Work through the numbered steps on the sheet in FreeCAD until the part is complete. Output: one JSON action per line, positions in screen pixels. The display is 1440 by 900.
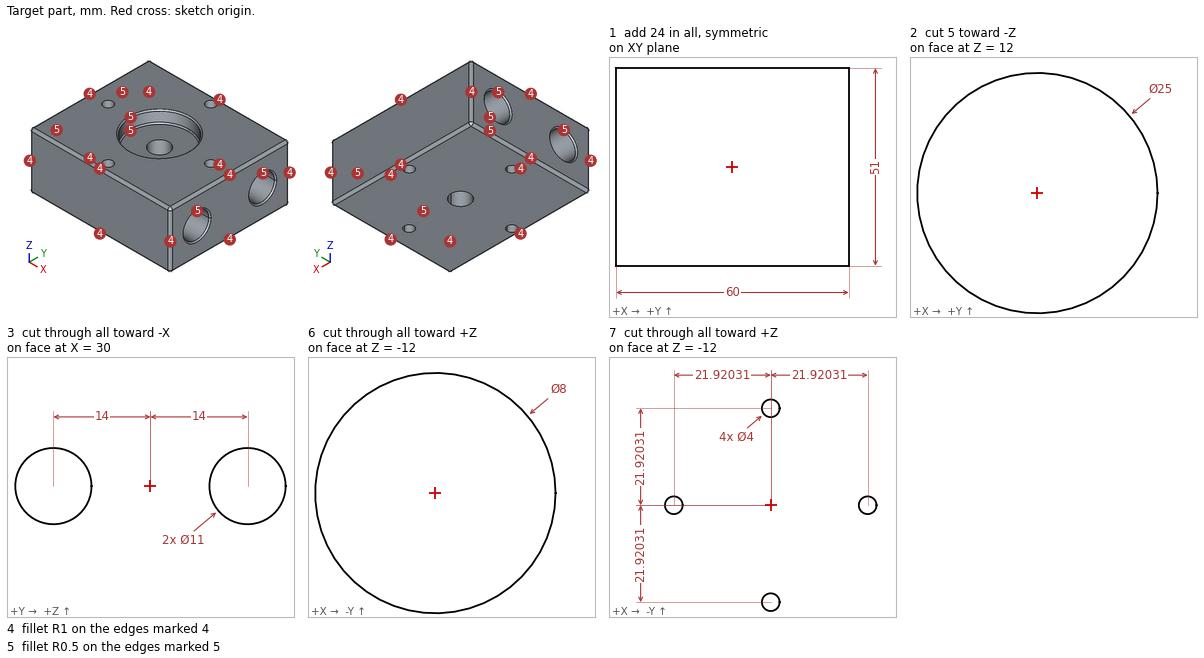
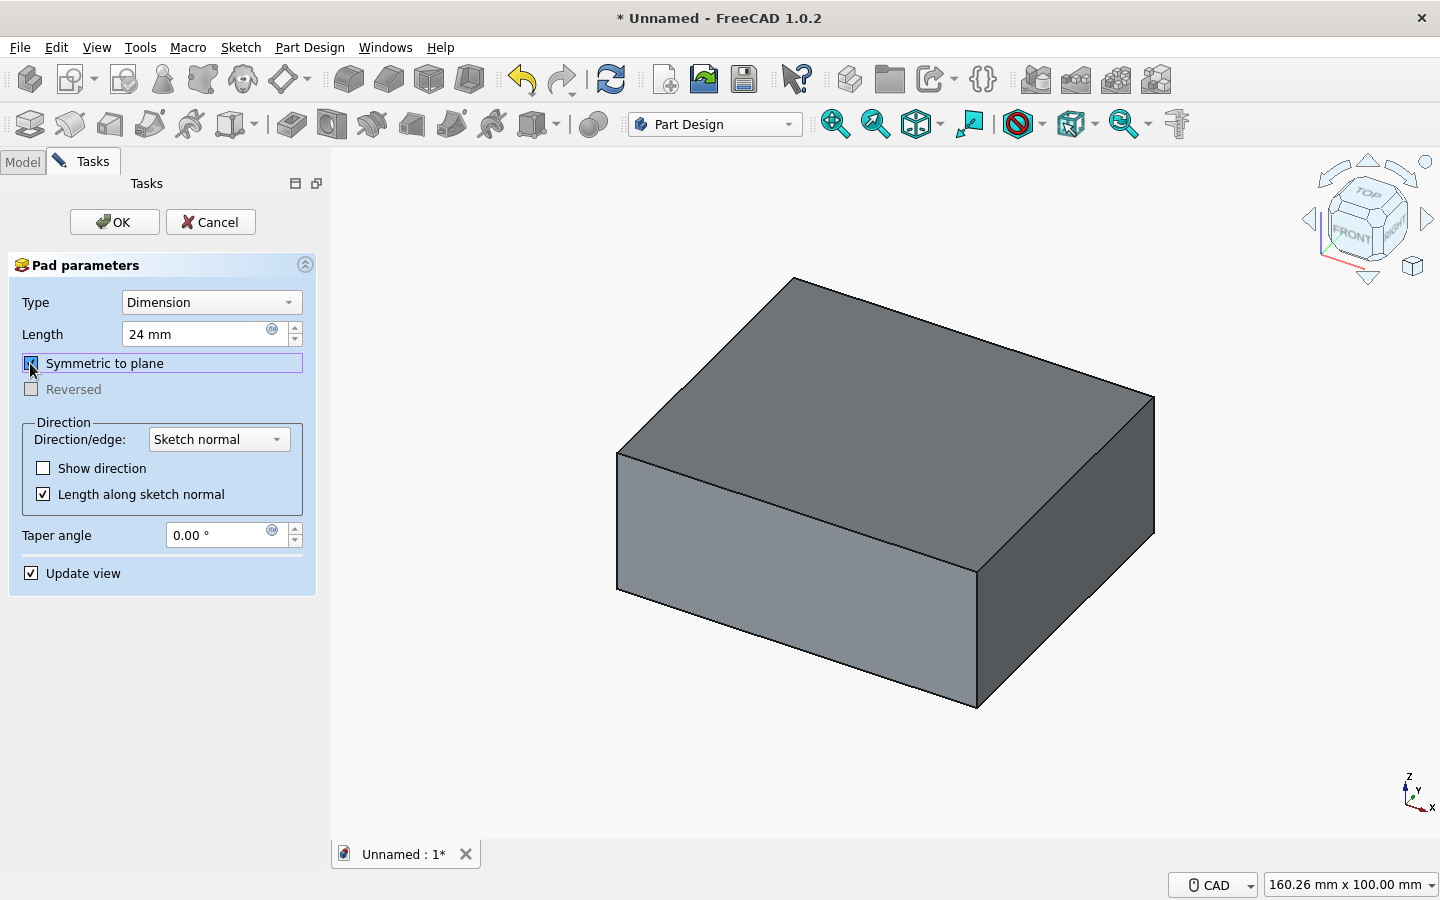
{"action": "left_click", "coordinate": [115, 222]}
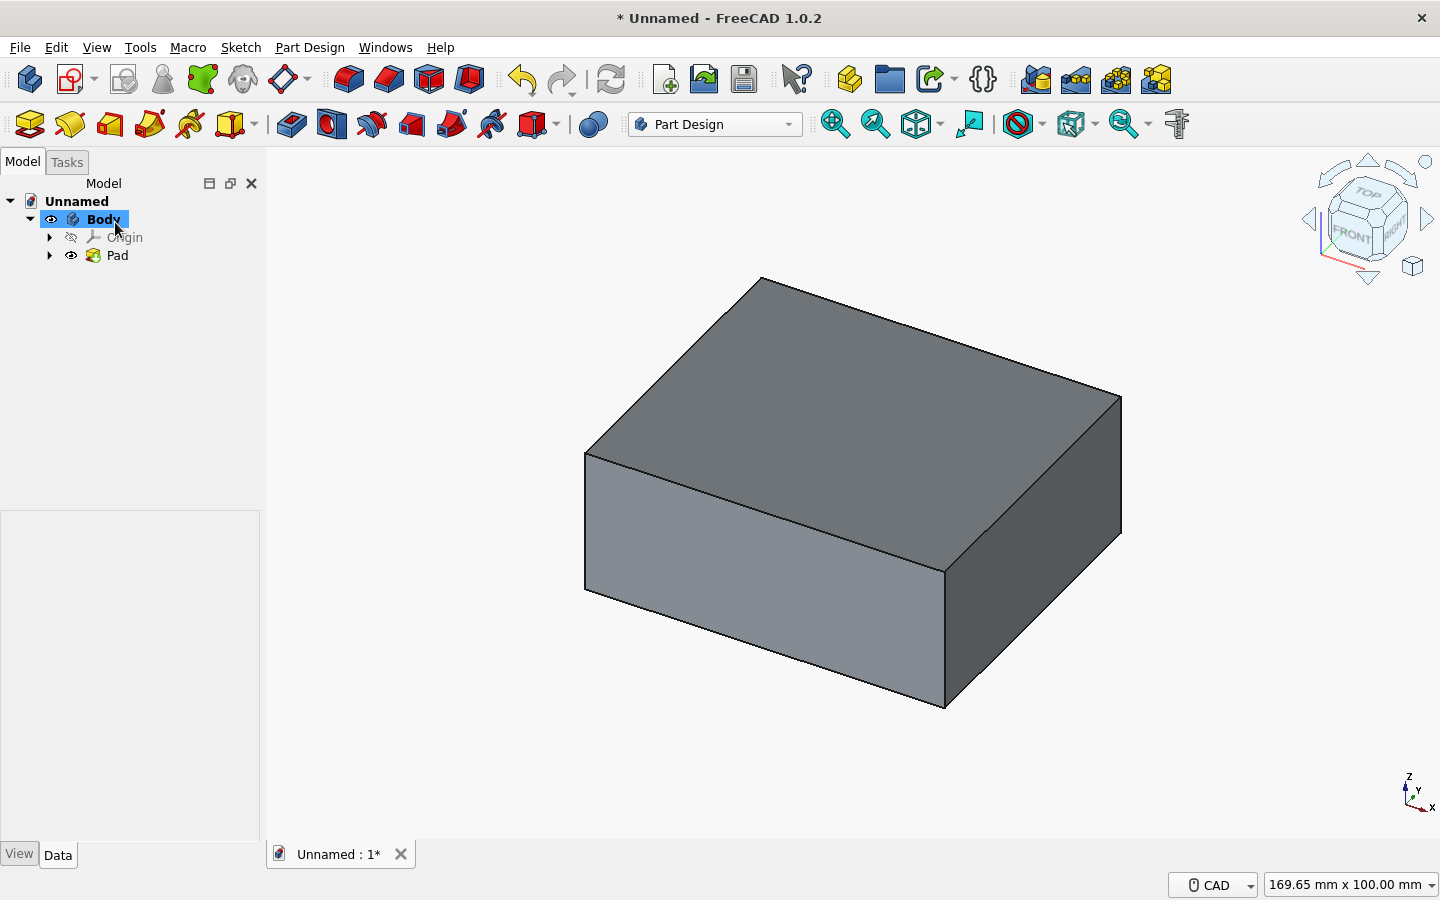
{"action": "left_click", "coordinate": [853, 424]}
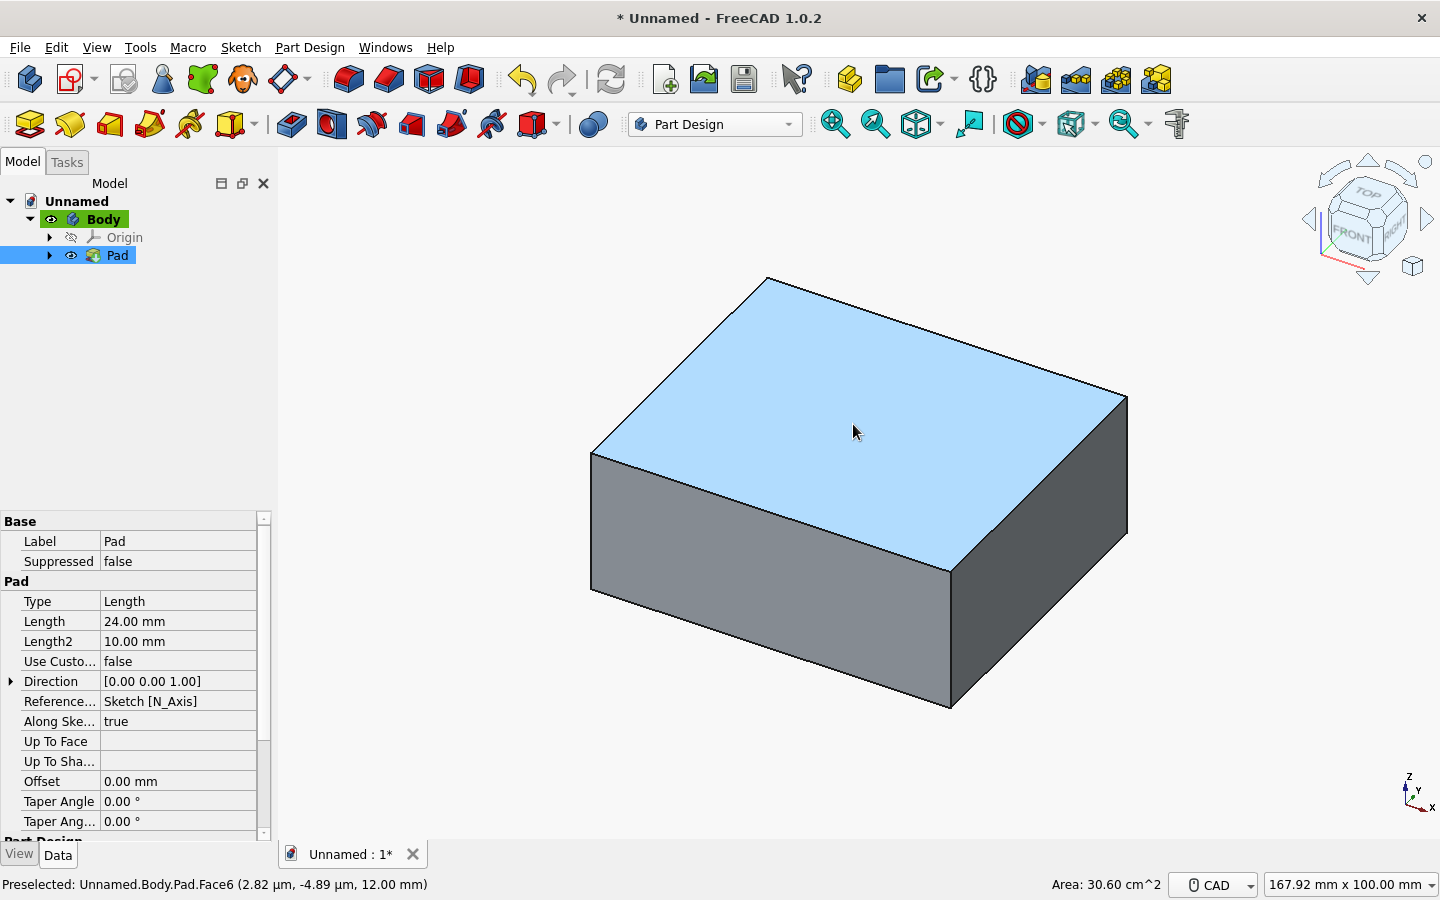
{"action": "left_click", "coordinate": [70, 80]}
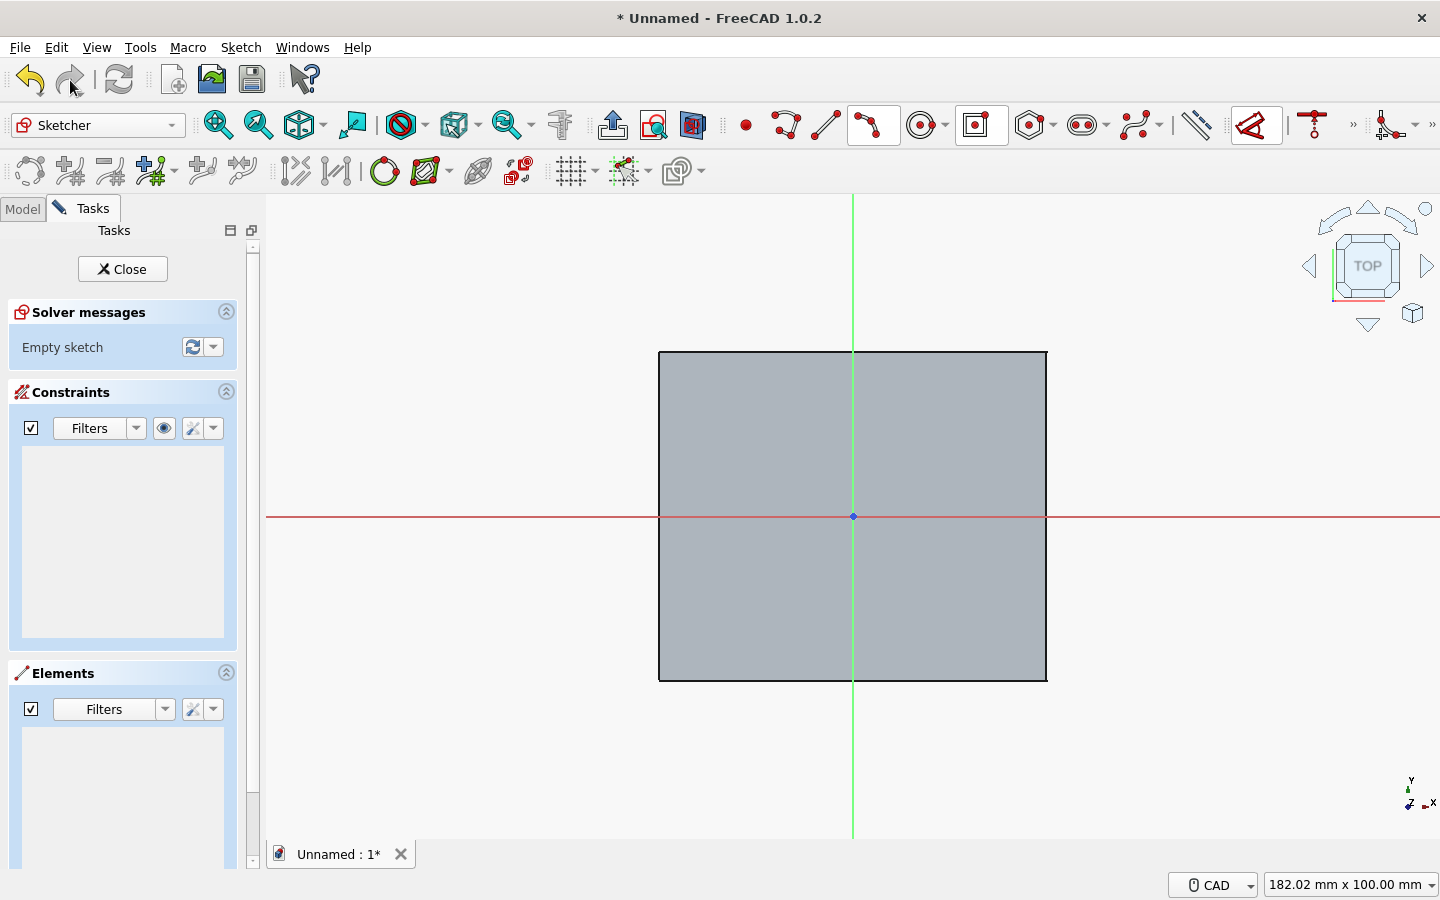
{"action": "scroll", "coordinate": [893, 516], "scroll_direction": "up", "scroll_amount": 5}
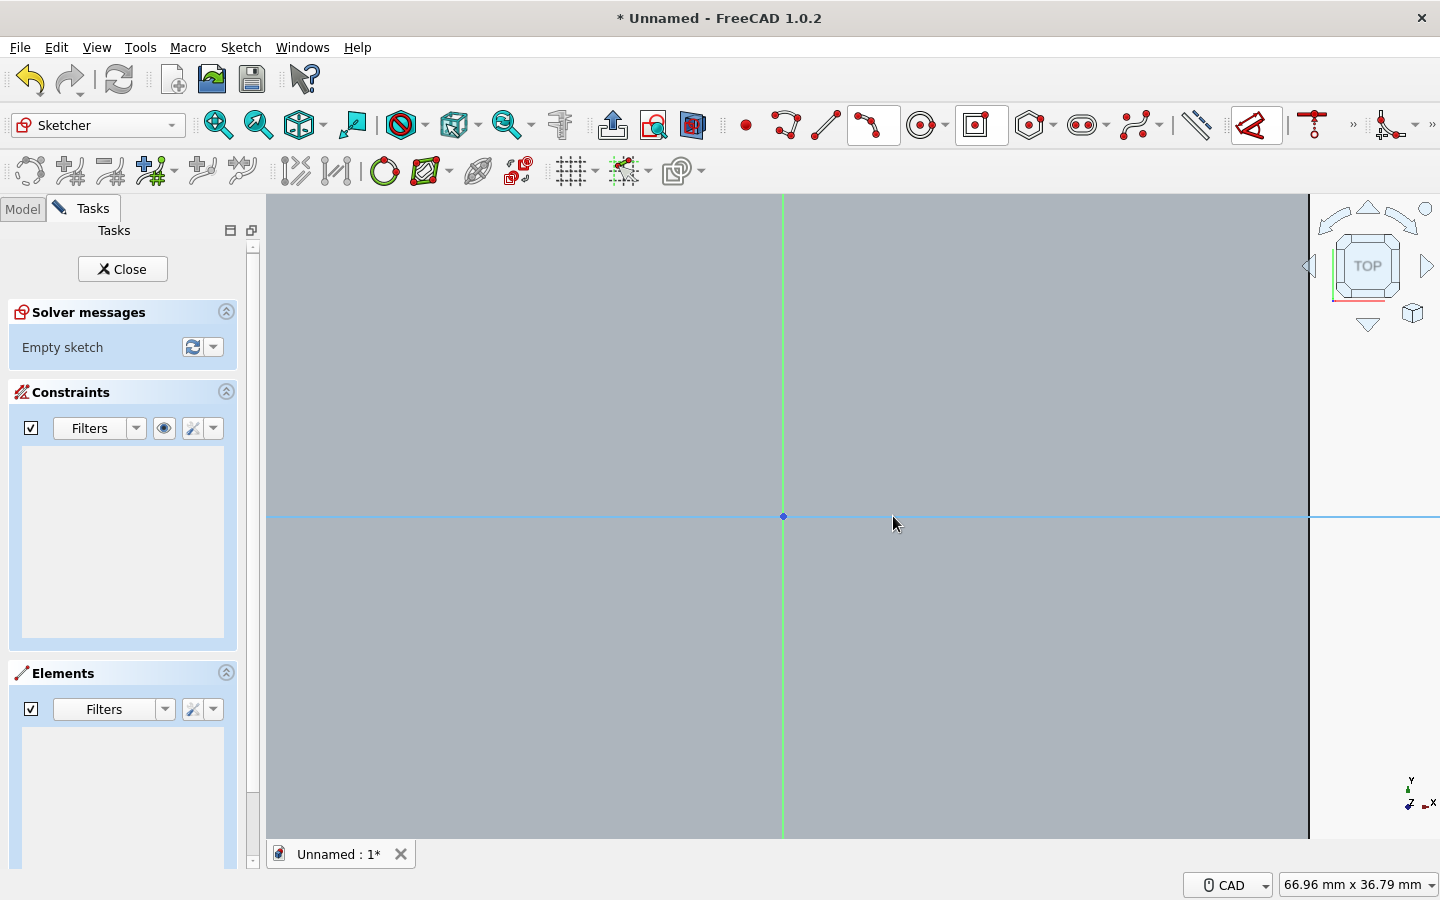
{"action": "key", "text": "g c"}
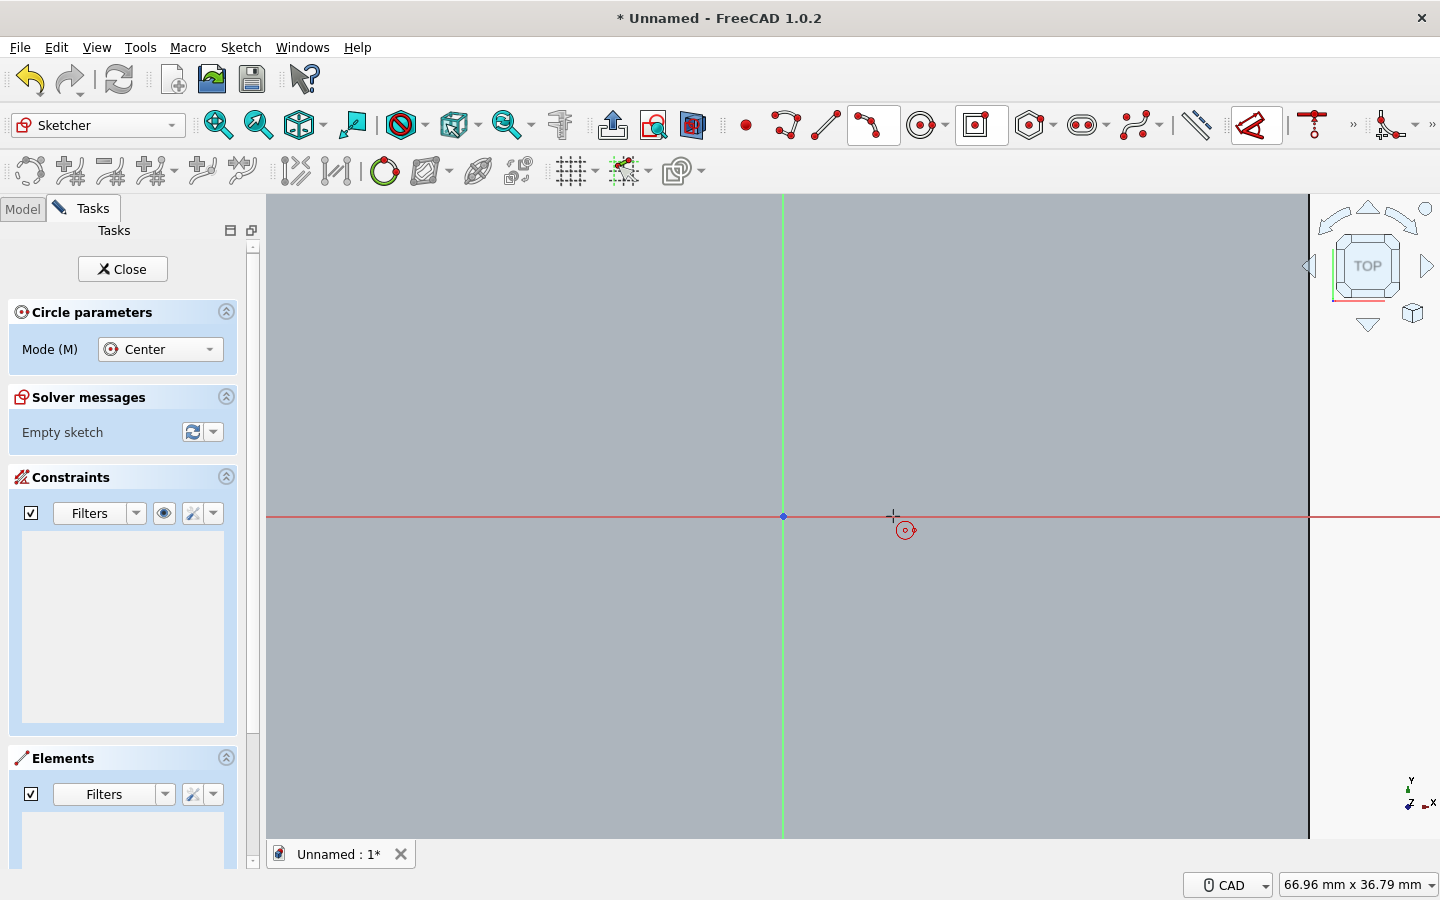
{"action": "left_click", "coordinate": [783, 516]}
{"action": "left_click", "coordinate": [938, 362]}
{"action": "key", "text": "Escape"}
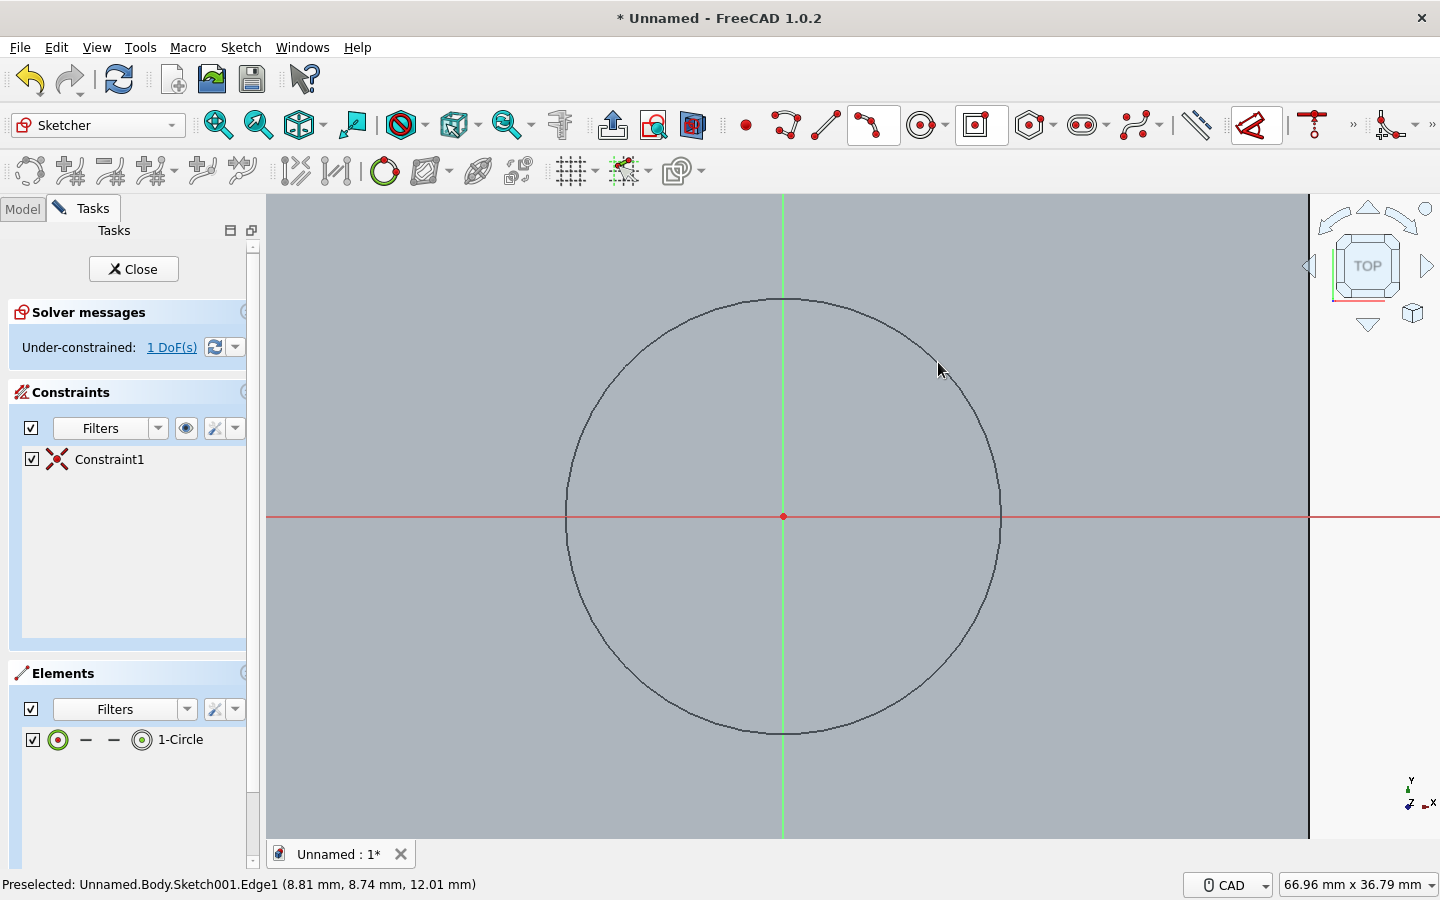
{"action": "left_click", "coordinate": [1250, 126]}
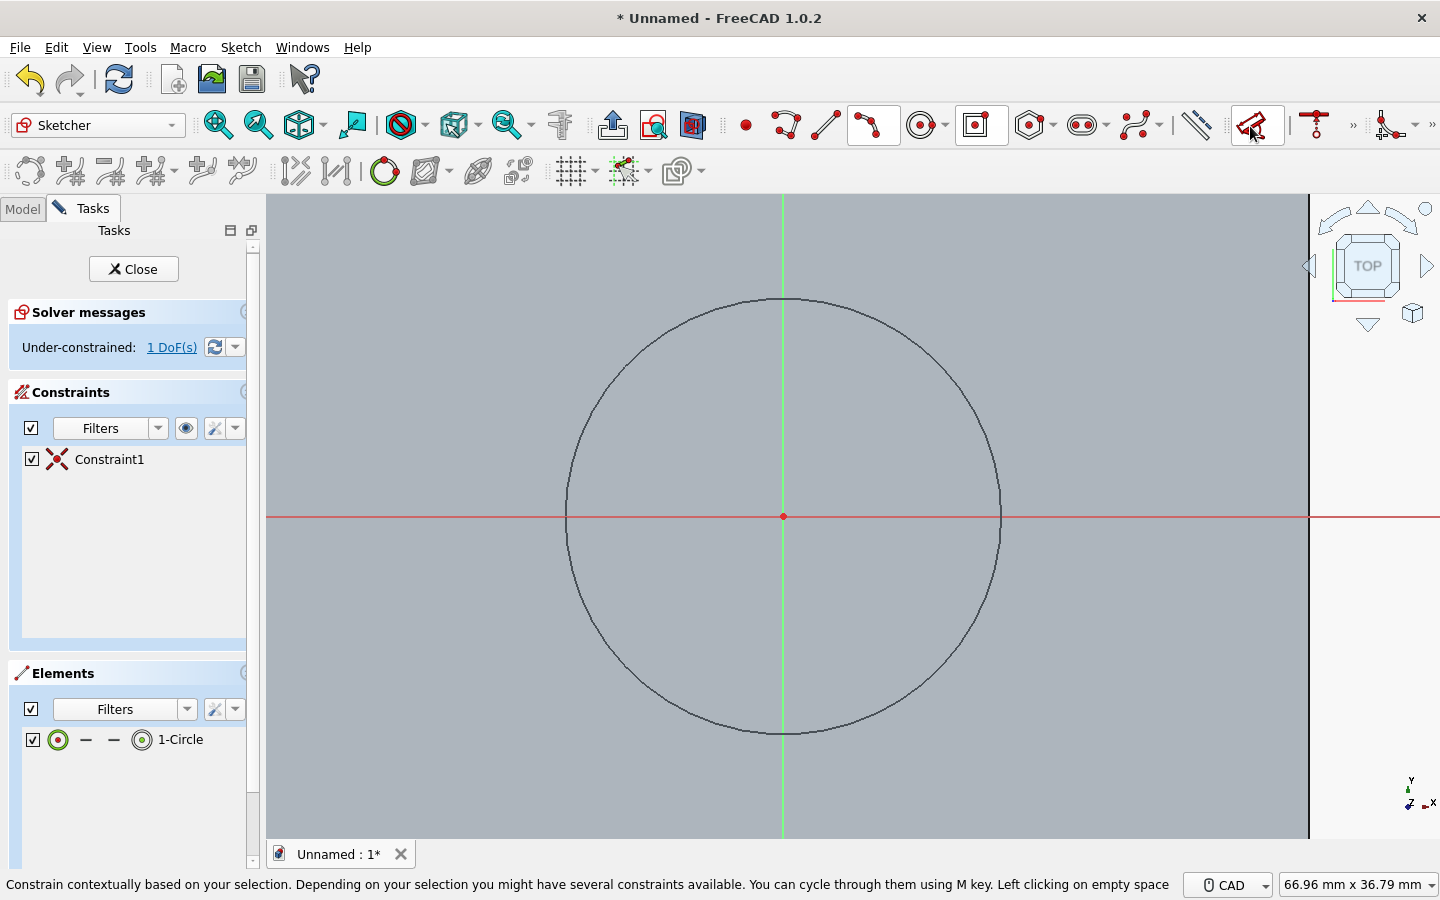
{"action": "left_click", "coordinate": [937, 362]}
{"action": "left_click", "coordinate": [960, 339]}